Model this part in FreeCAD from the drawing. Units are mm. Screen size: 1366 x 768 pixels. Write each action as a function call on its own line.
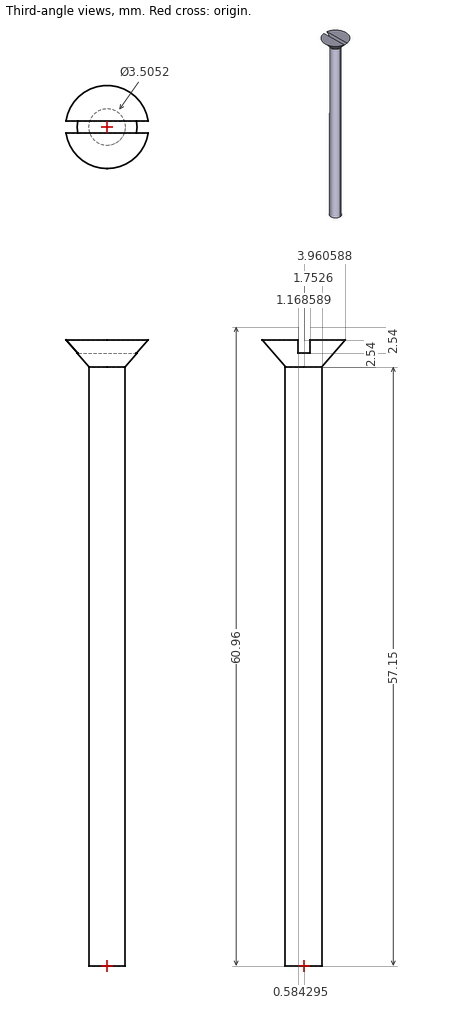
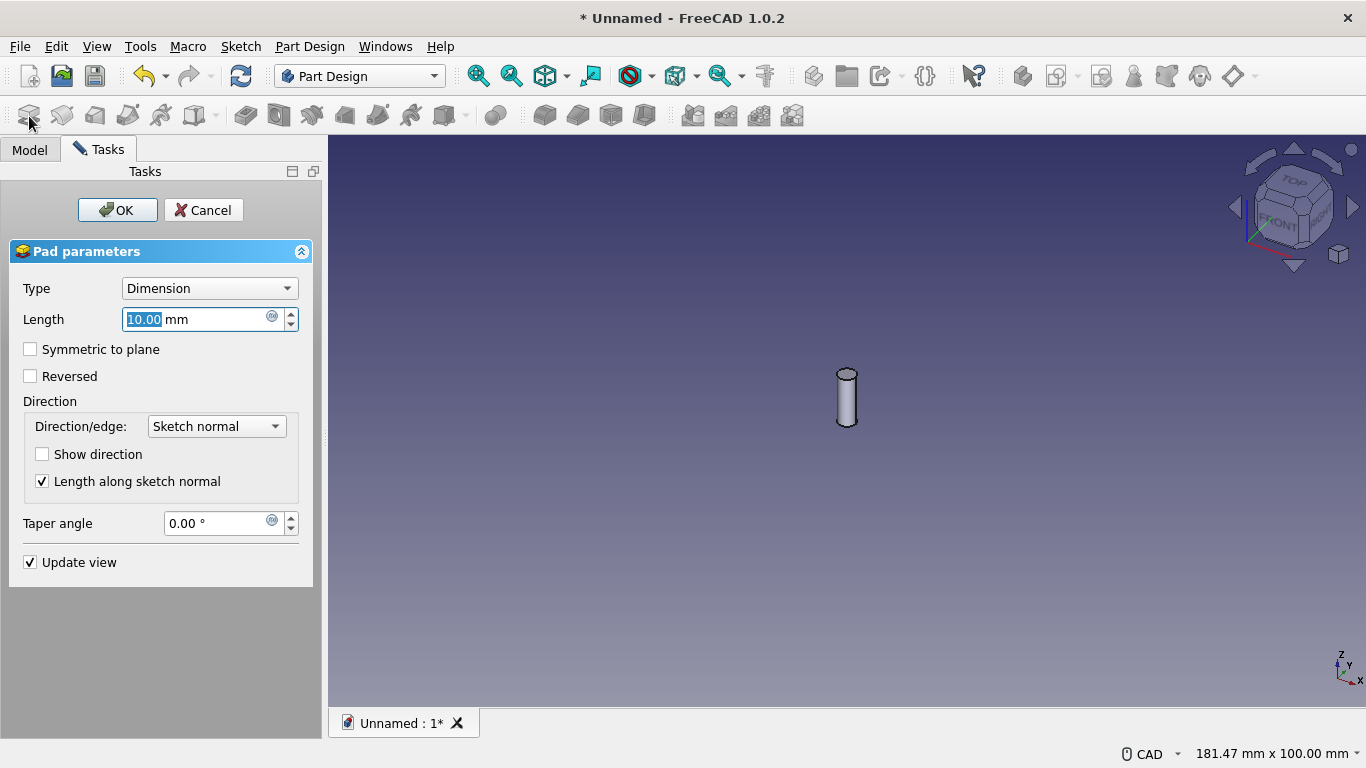
text(57.15)
key(Tab)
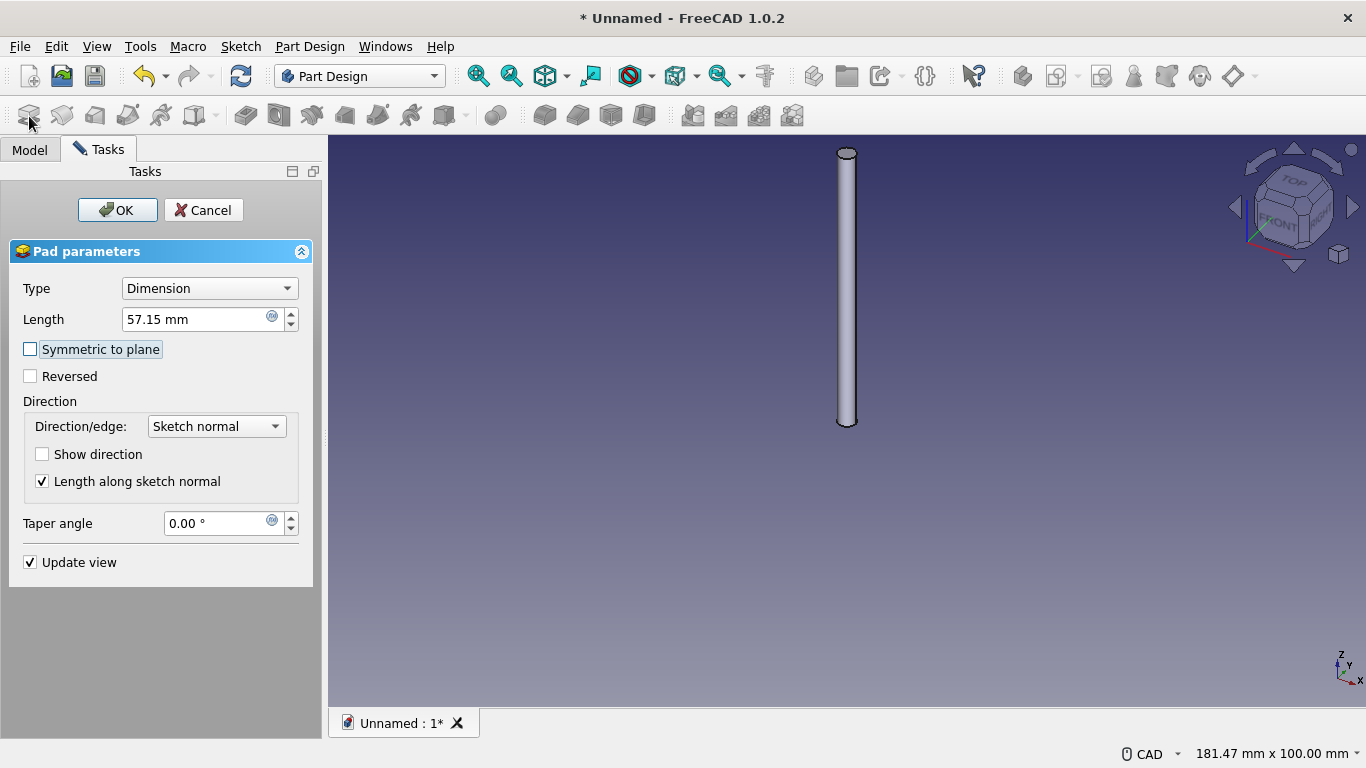
click(118, 210)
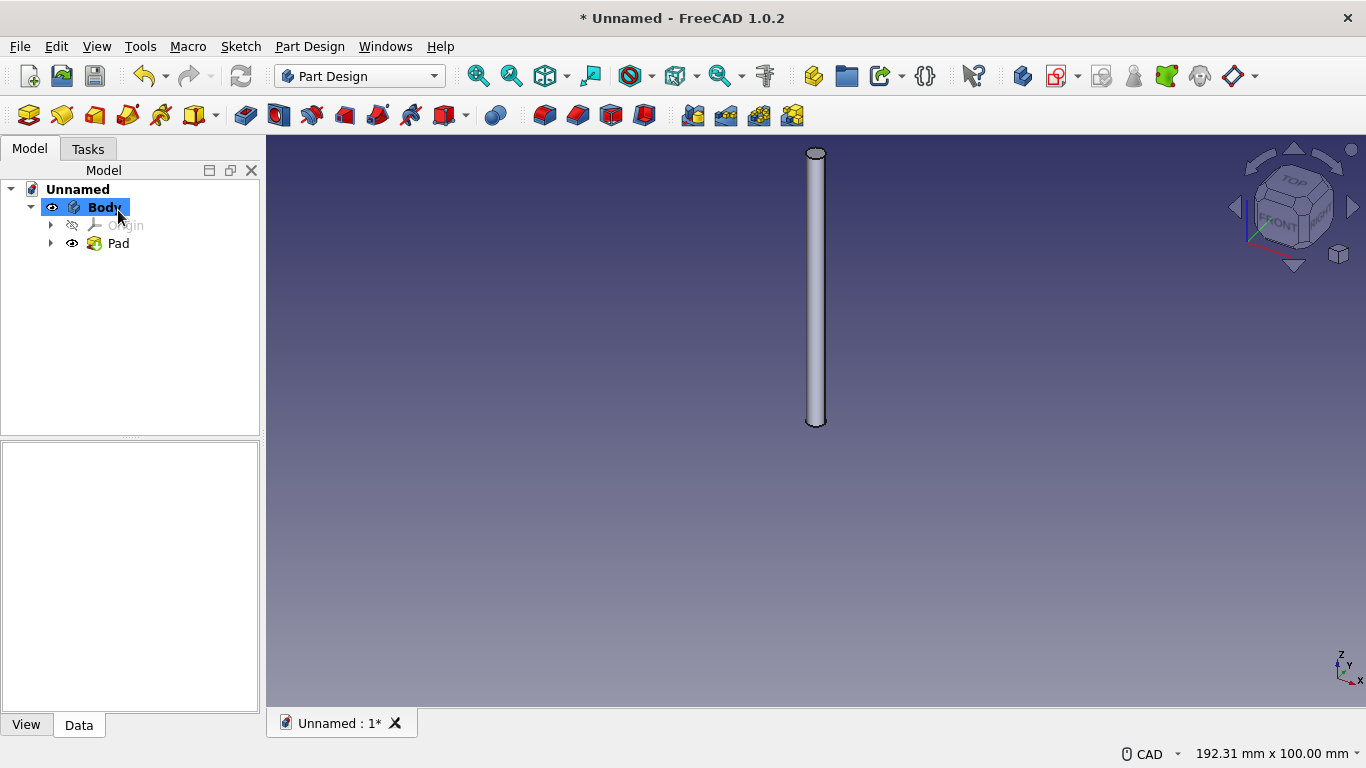
click(1056, 76)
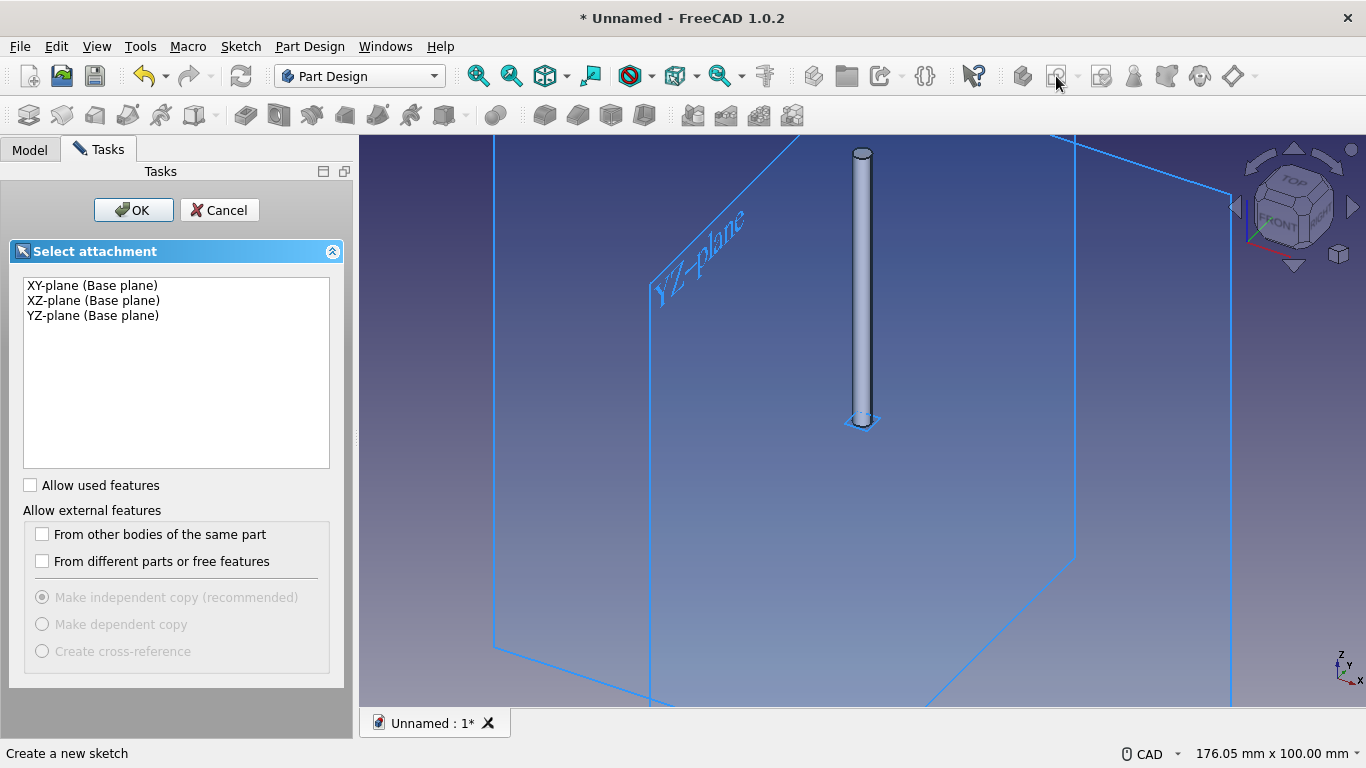
click(84, 316)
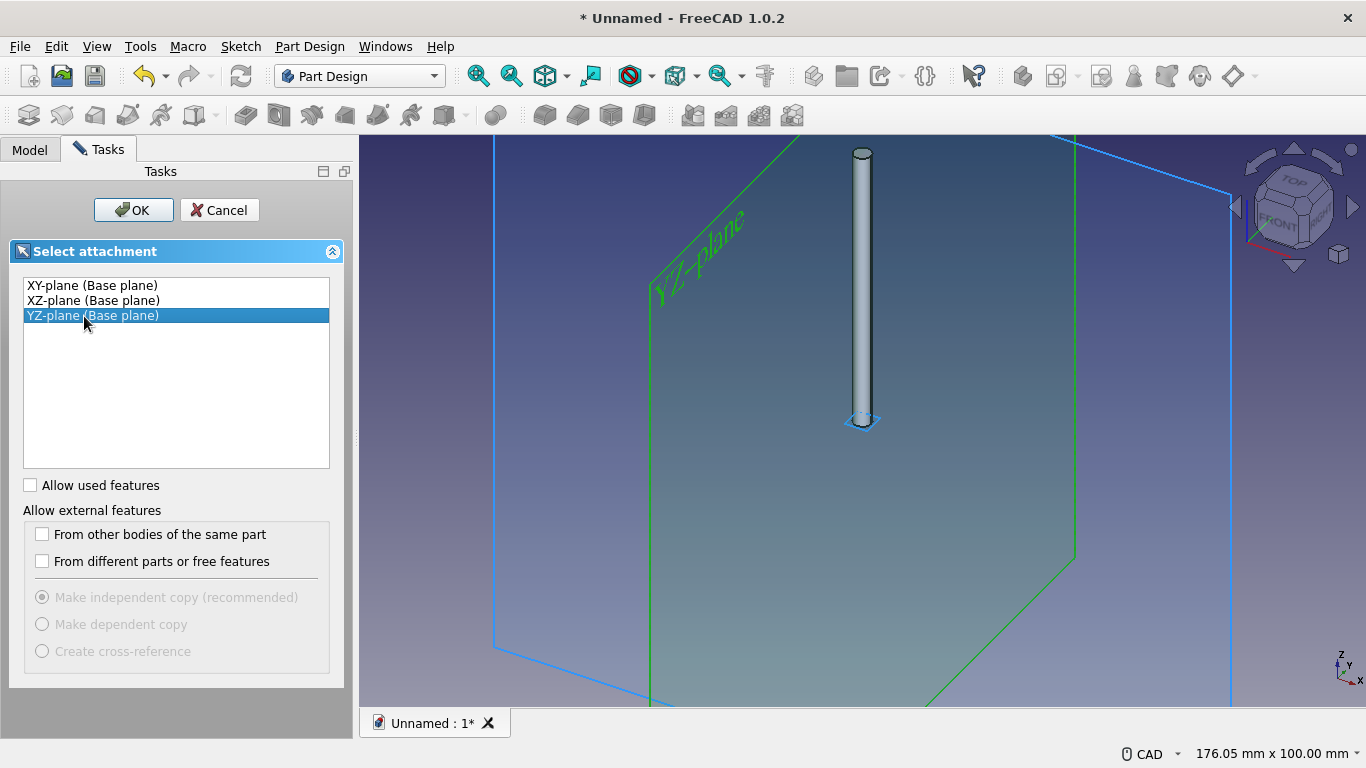
click(134, 210)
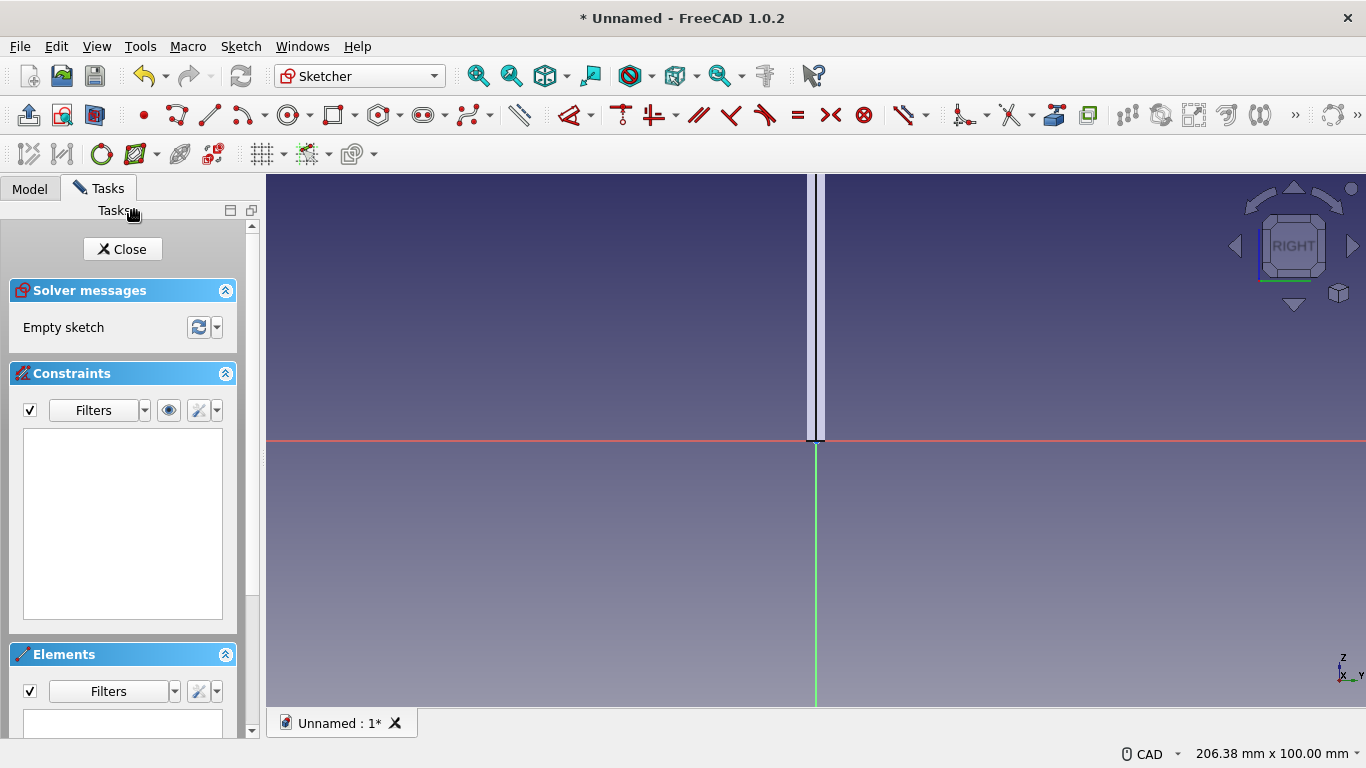
click(95, 116)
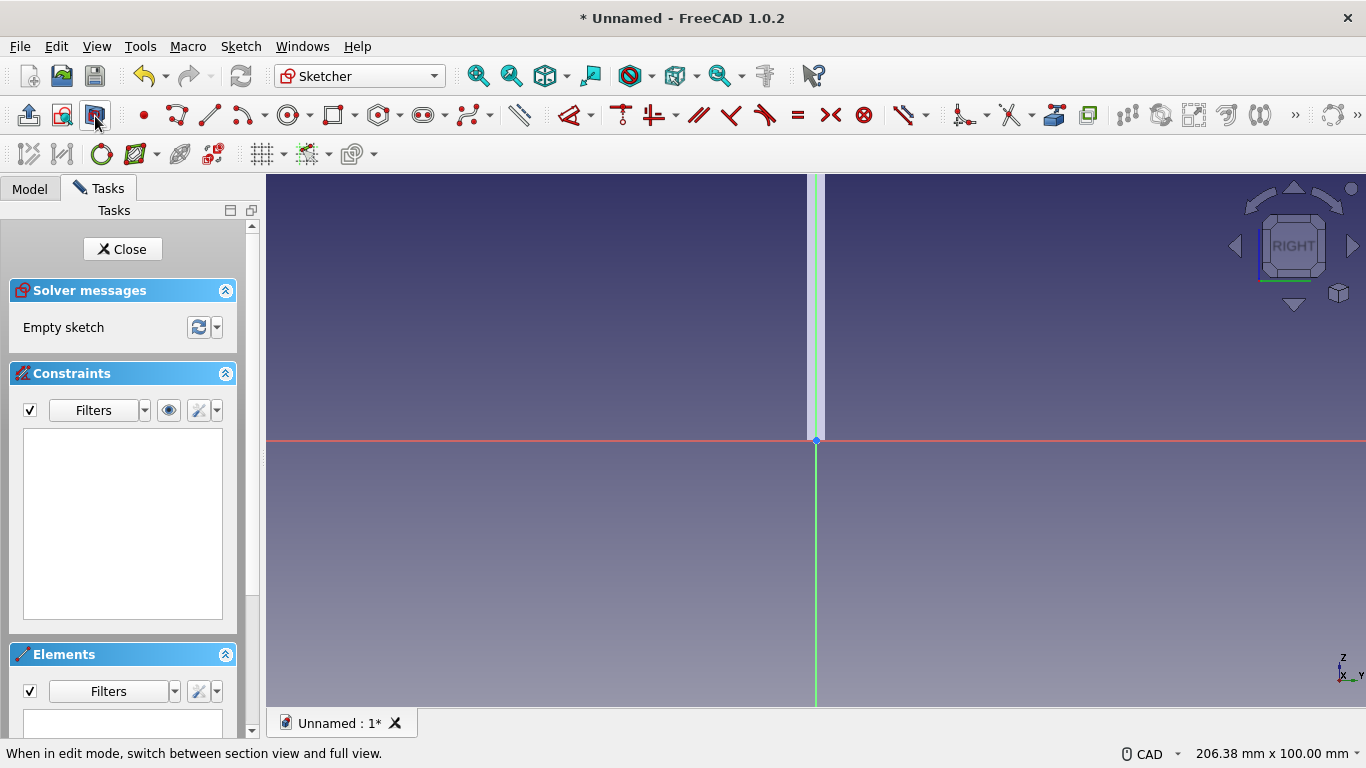
scroll(748, 440, down, 5)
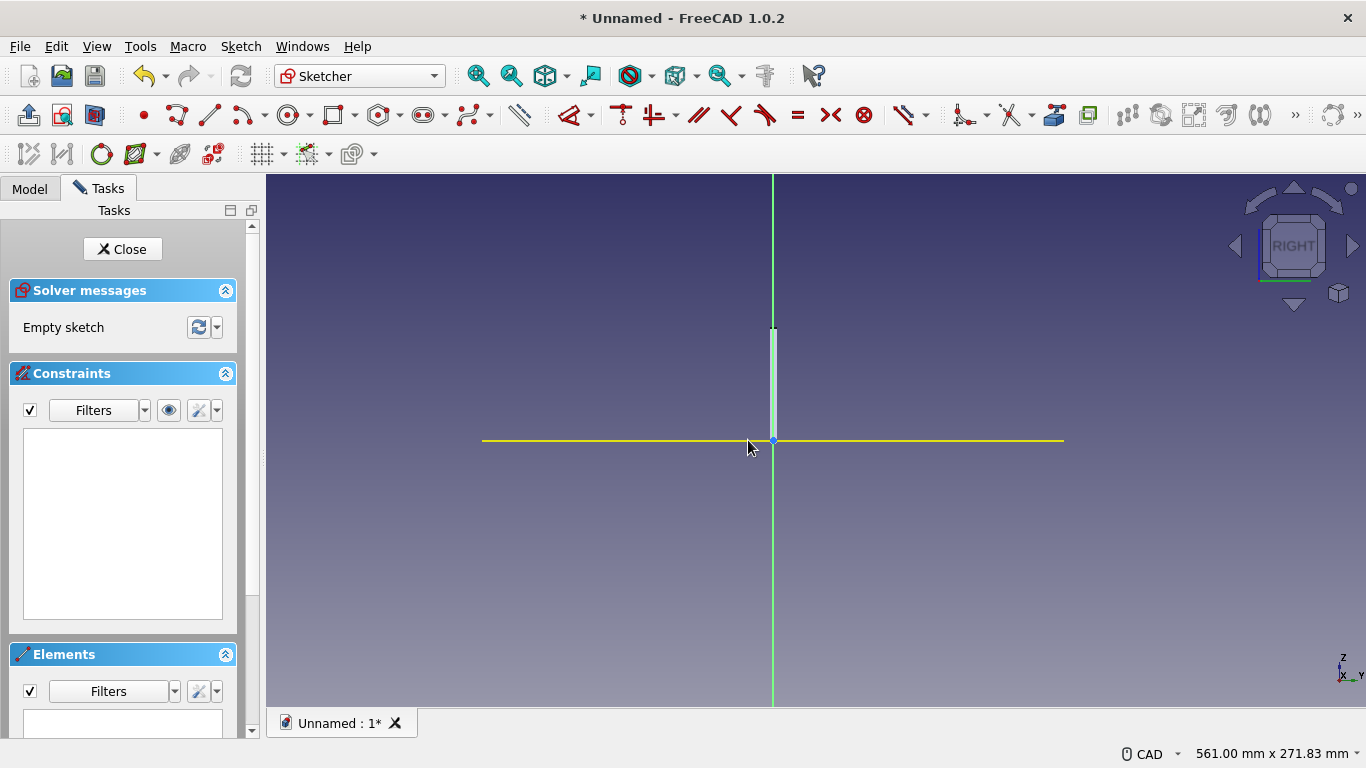
scroll(779, 320, up, 15)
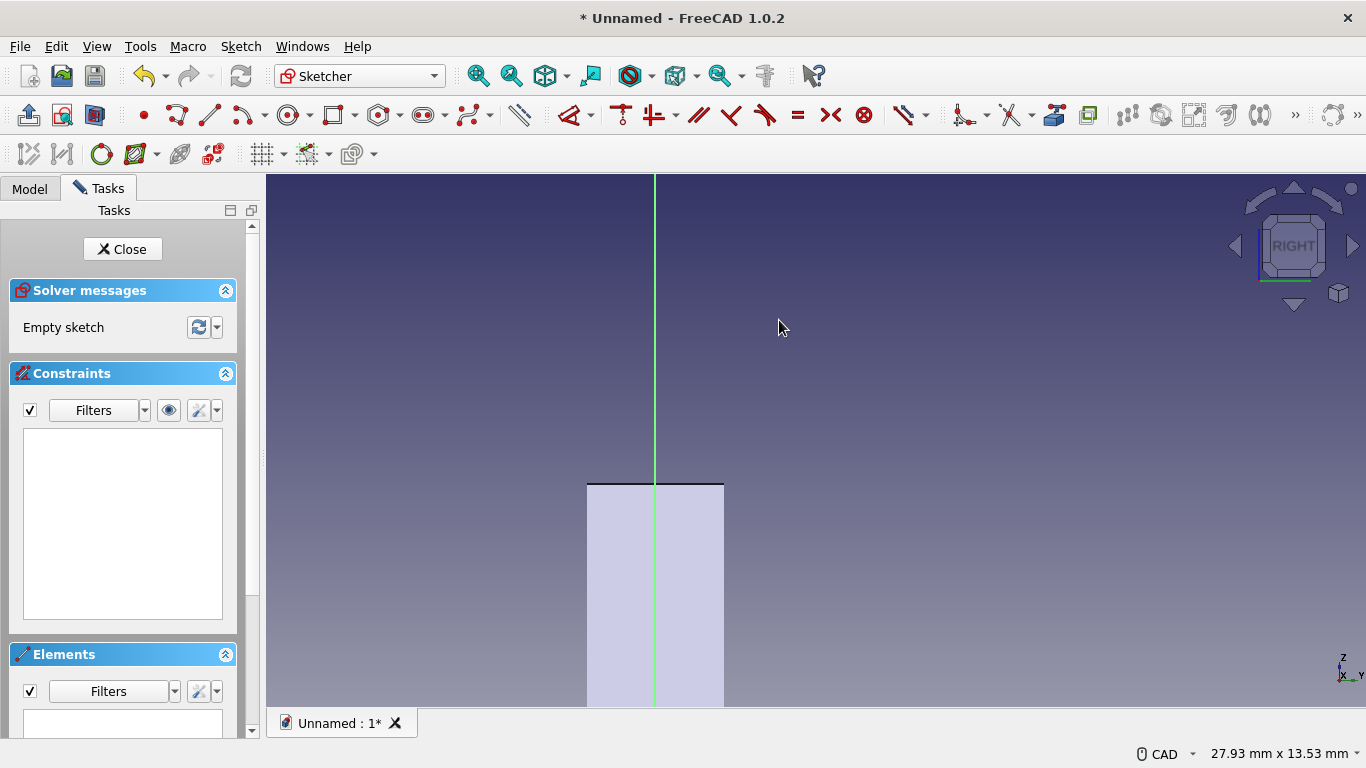
scroll(727, 432, up, 6)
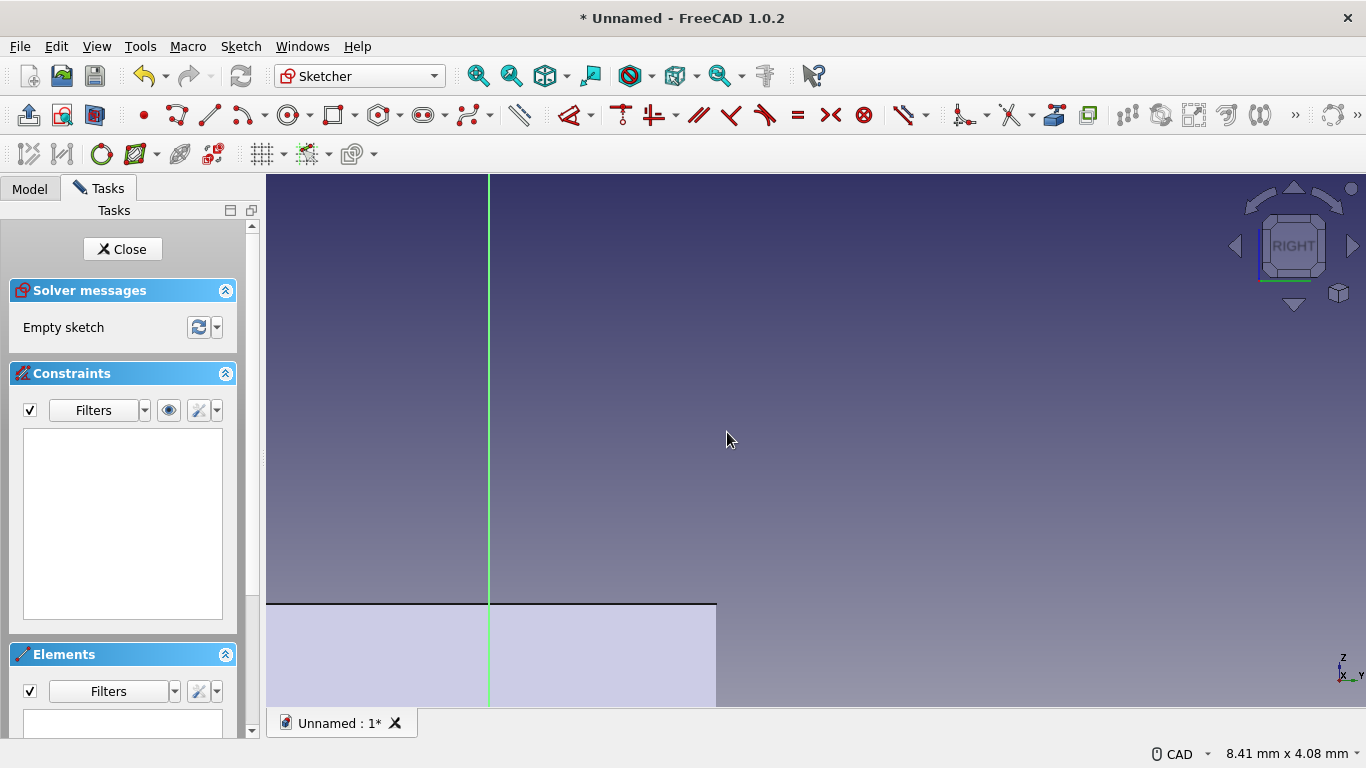
click(177, 116)